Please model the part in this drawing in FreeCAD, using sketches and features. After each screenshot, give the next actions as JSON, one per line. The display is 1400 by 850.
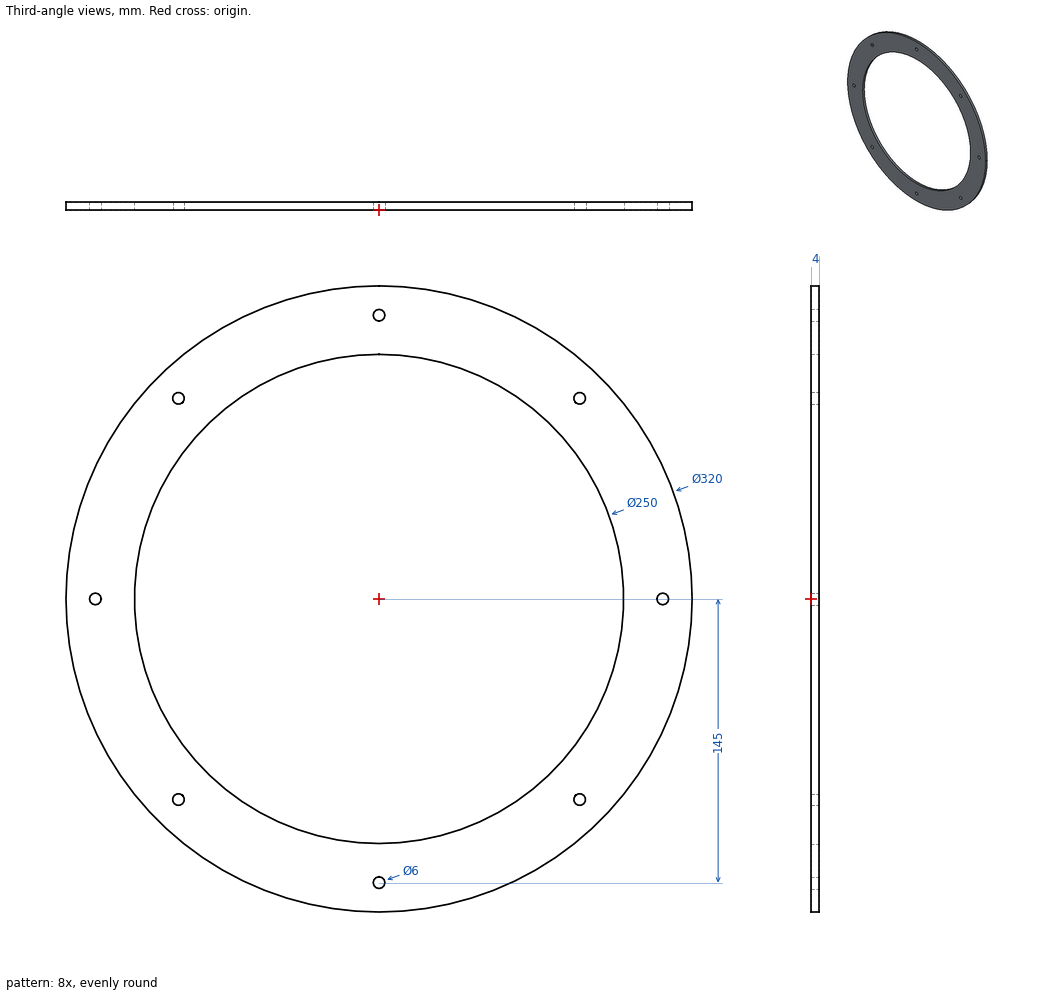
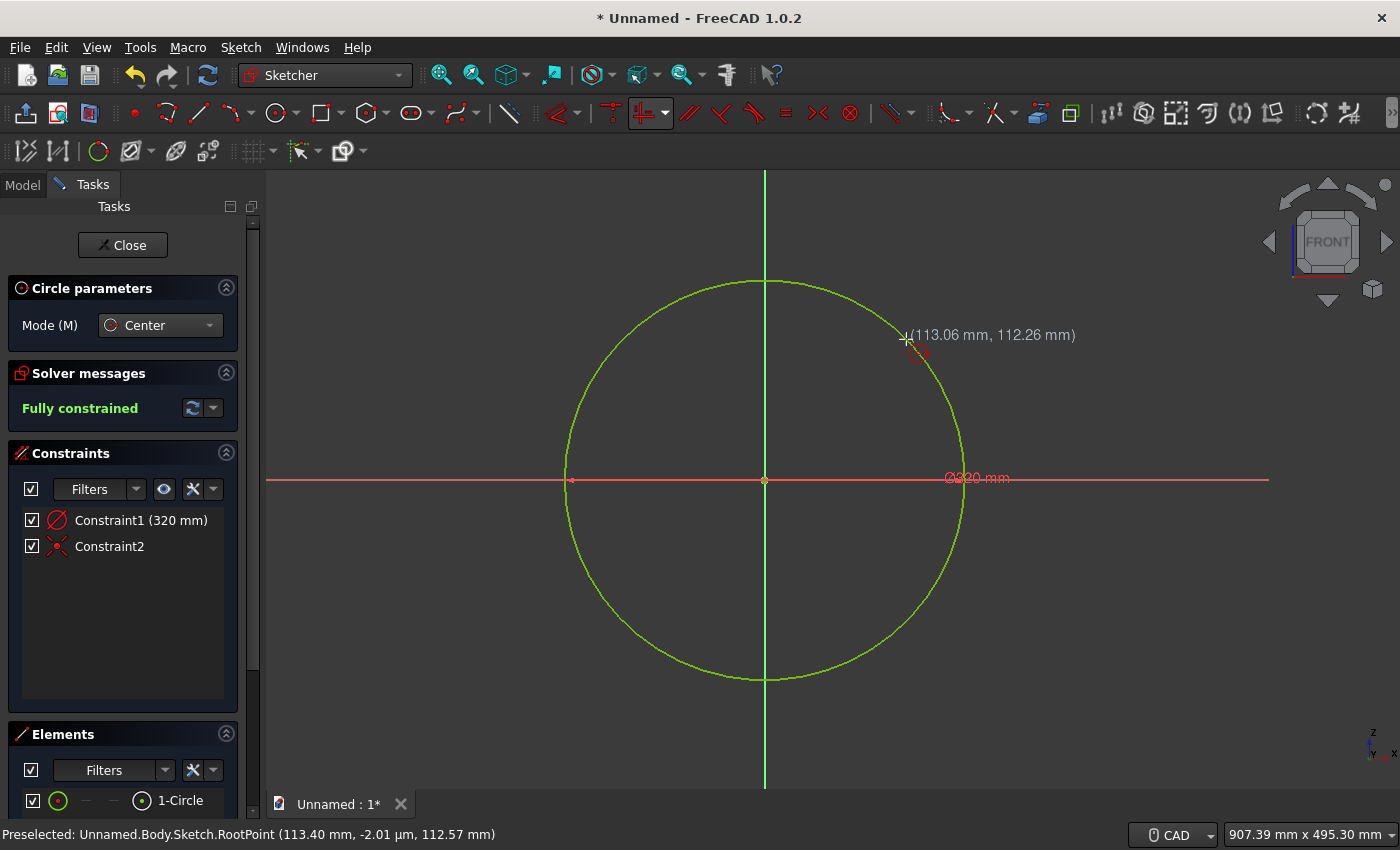
{"action": "left_click", "coordinate": [765, 480]}
{"action": "mouse_move", "coordinate": [875, 370]}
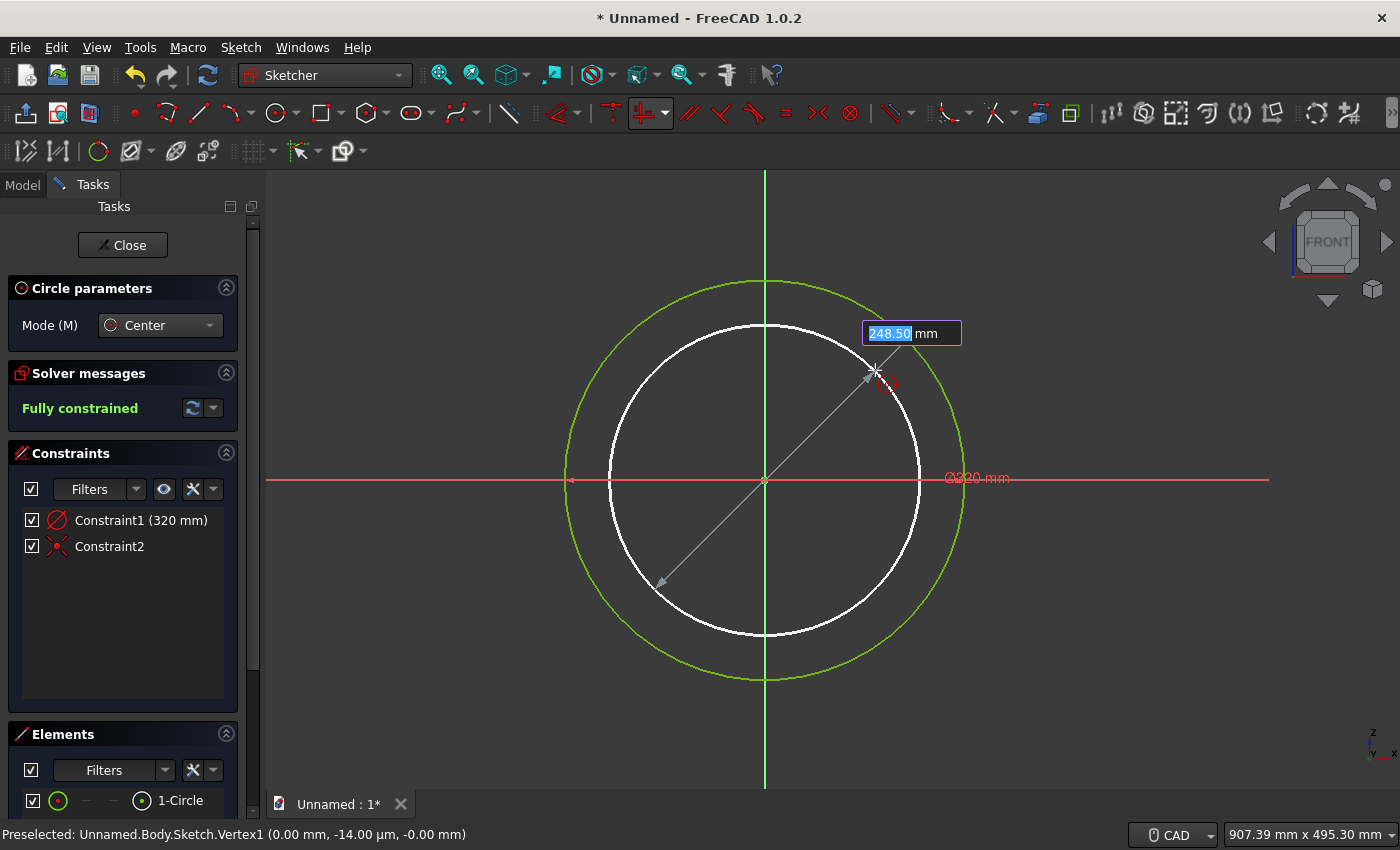
{"action": "type", "text": "250"}
{"action": "key", "text": "Return"}
{"action": "key", "text": "Escape"}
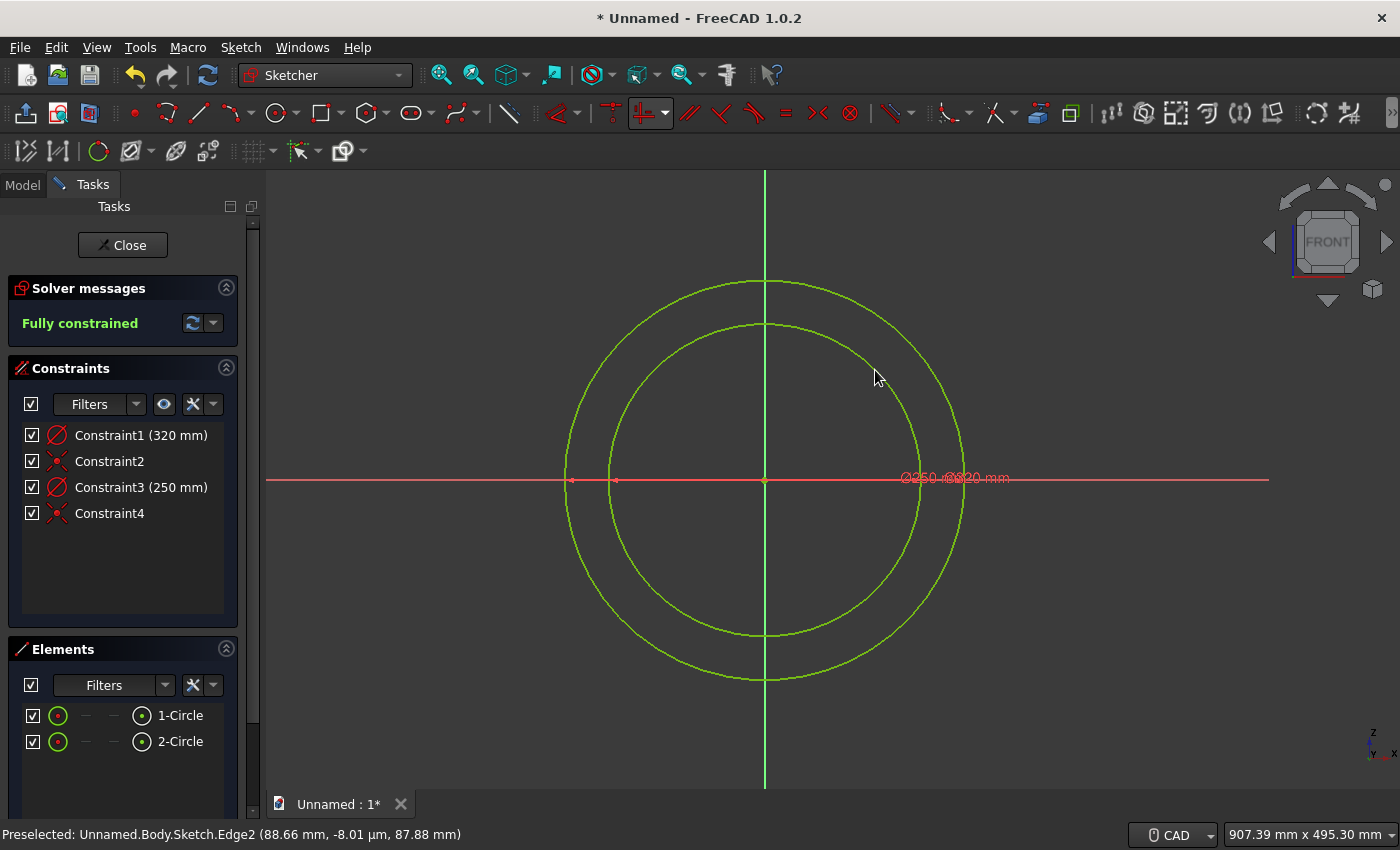
{"action": "left_click", "coordinate": [123, 245]}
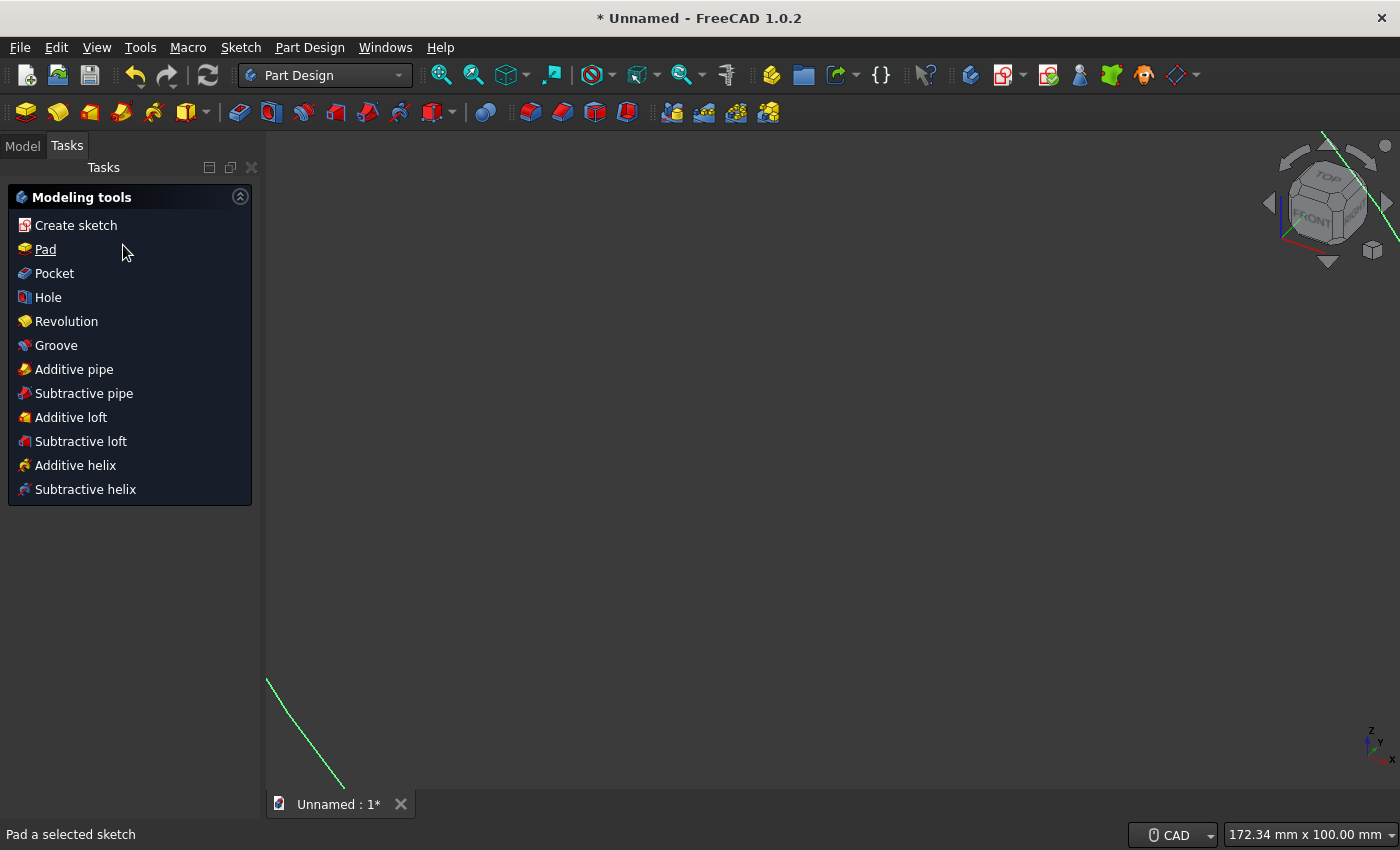
{"action": "left_click", "coordinate": [26, 112]}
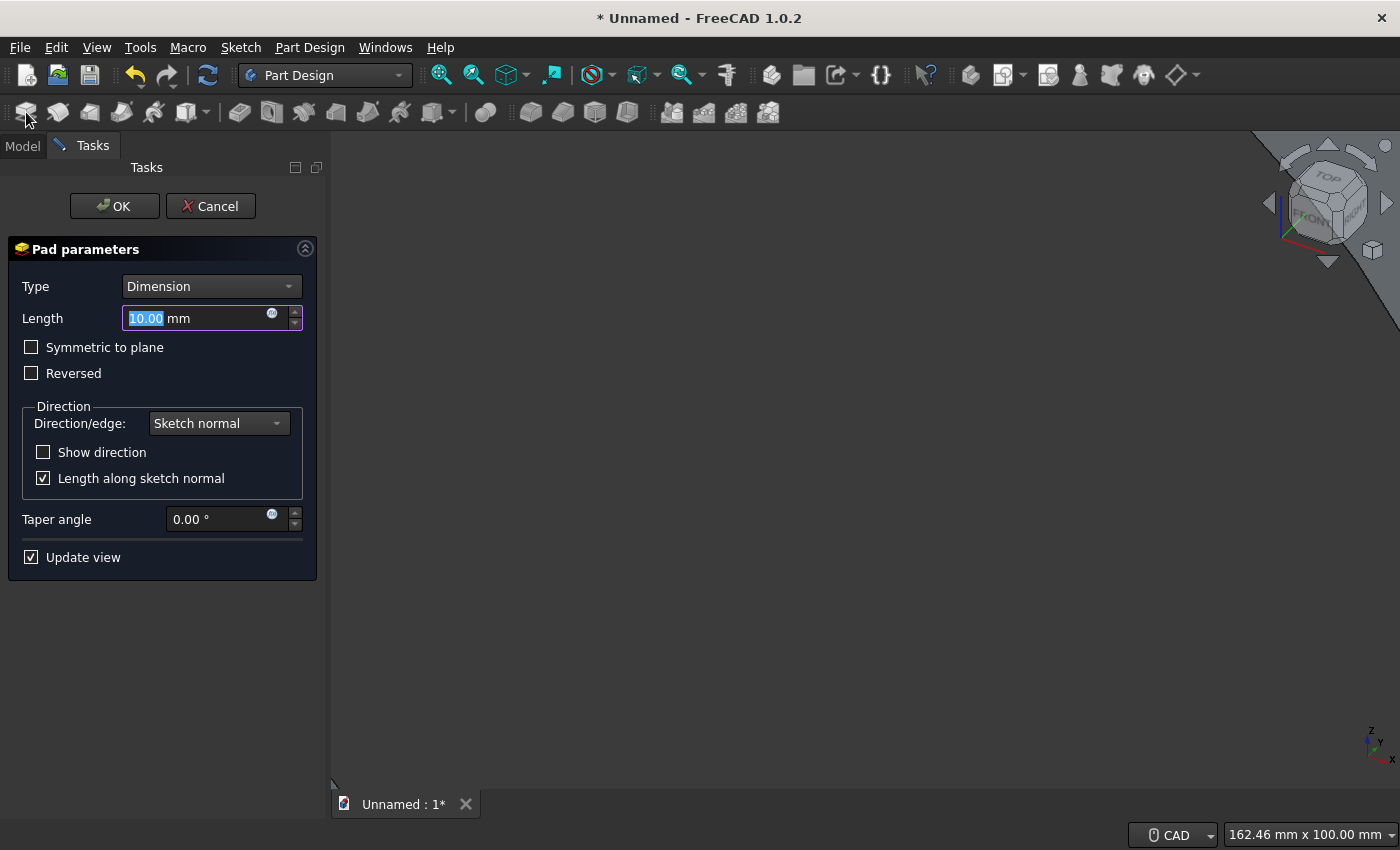
{"action": "type", "text": "4"}
{"action": "key", "text": "Tab"}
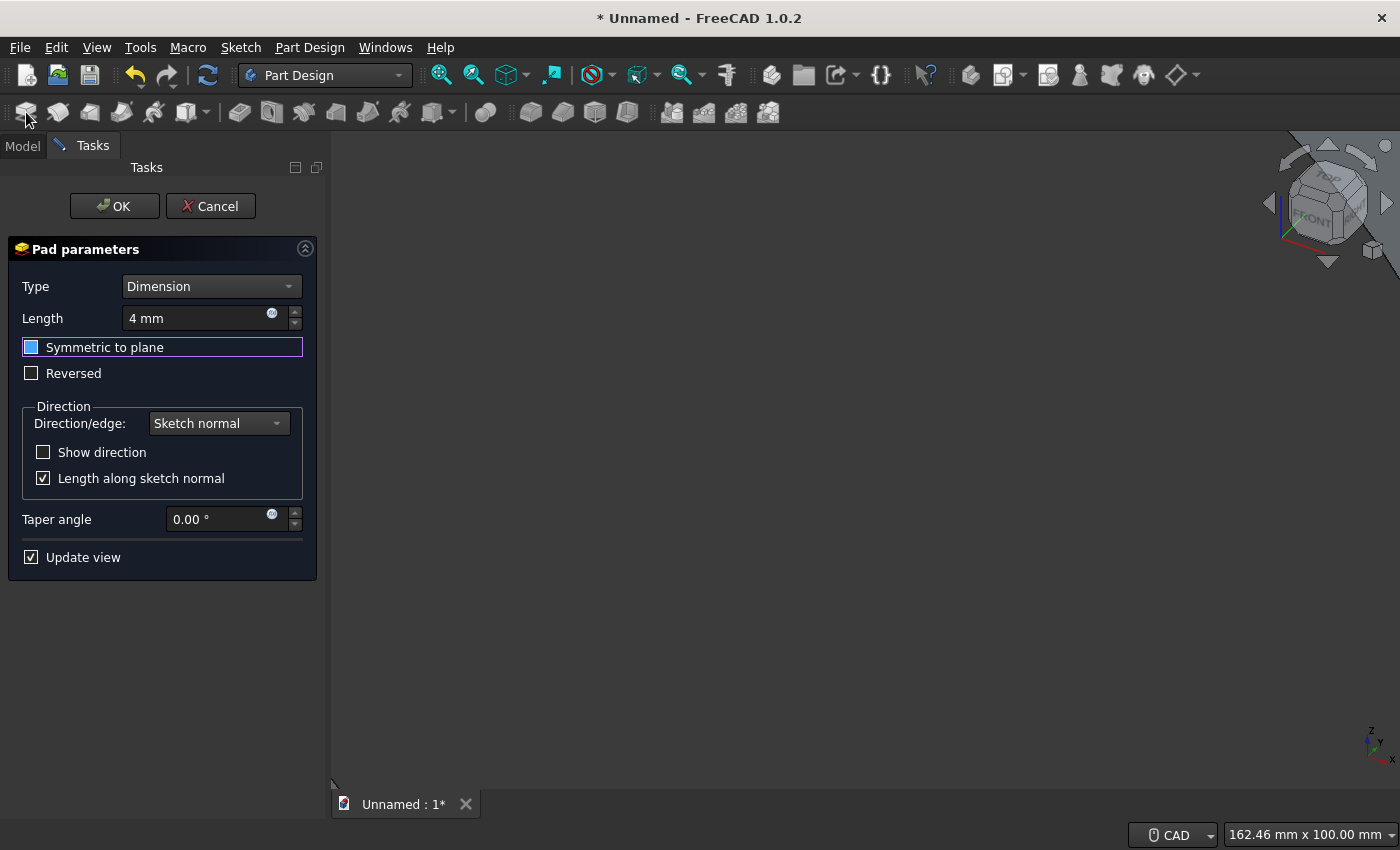
{"action": "left_click", "coordinate": [30, 373]}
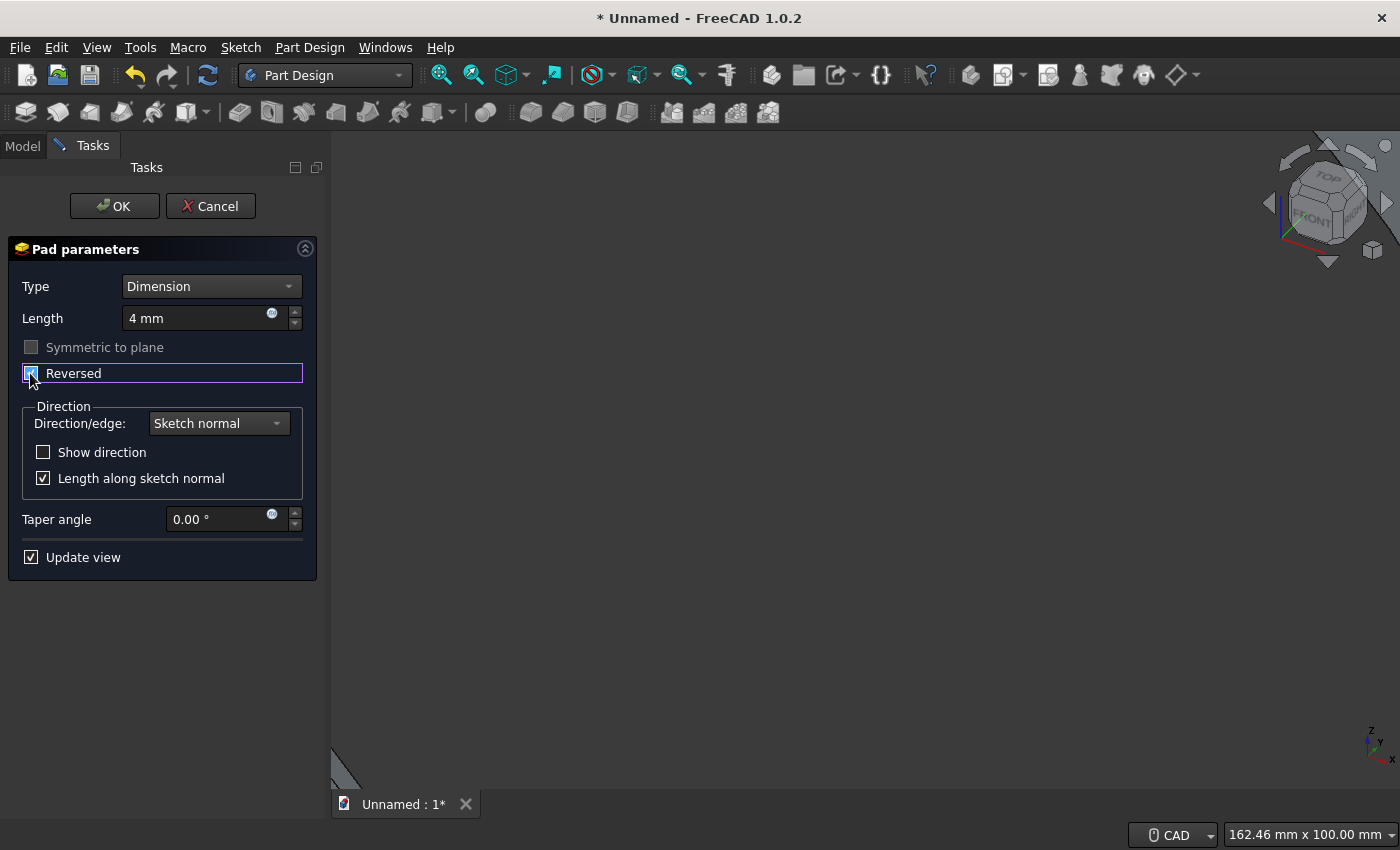
{"action": "left_click", "coordinate": [115, 206]}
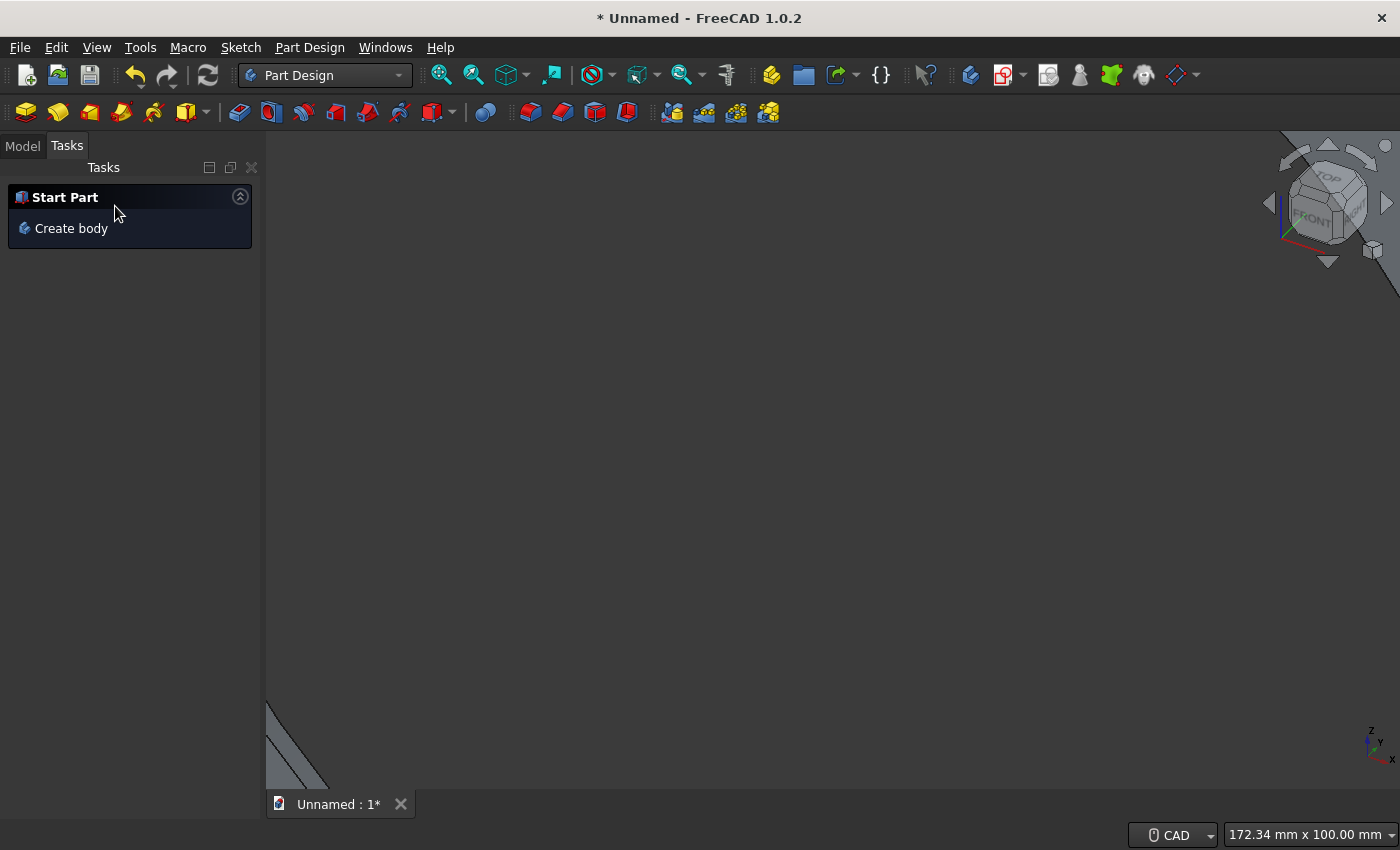
{"action": "key", "text": "v f"}